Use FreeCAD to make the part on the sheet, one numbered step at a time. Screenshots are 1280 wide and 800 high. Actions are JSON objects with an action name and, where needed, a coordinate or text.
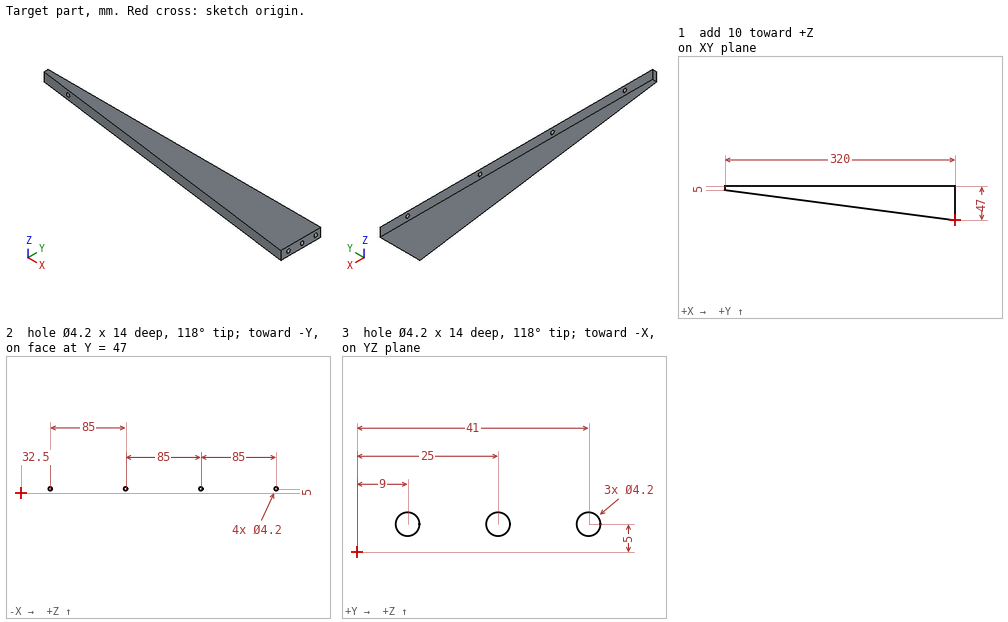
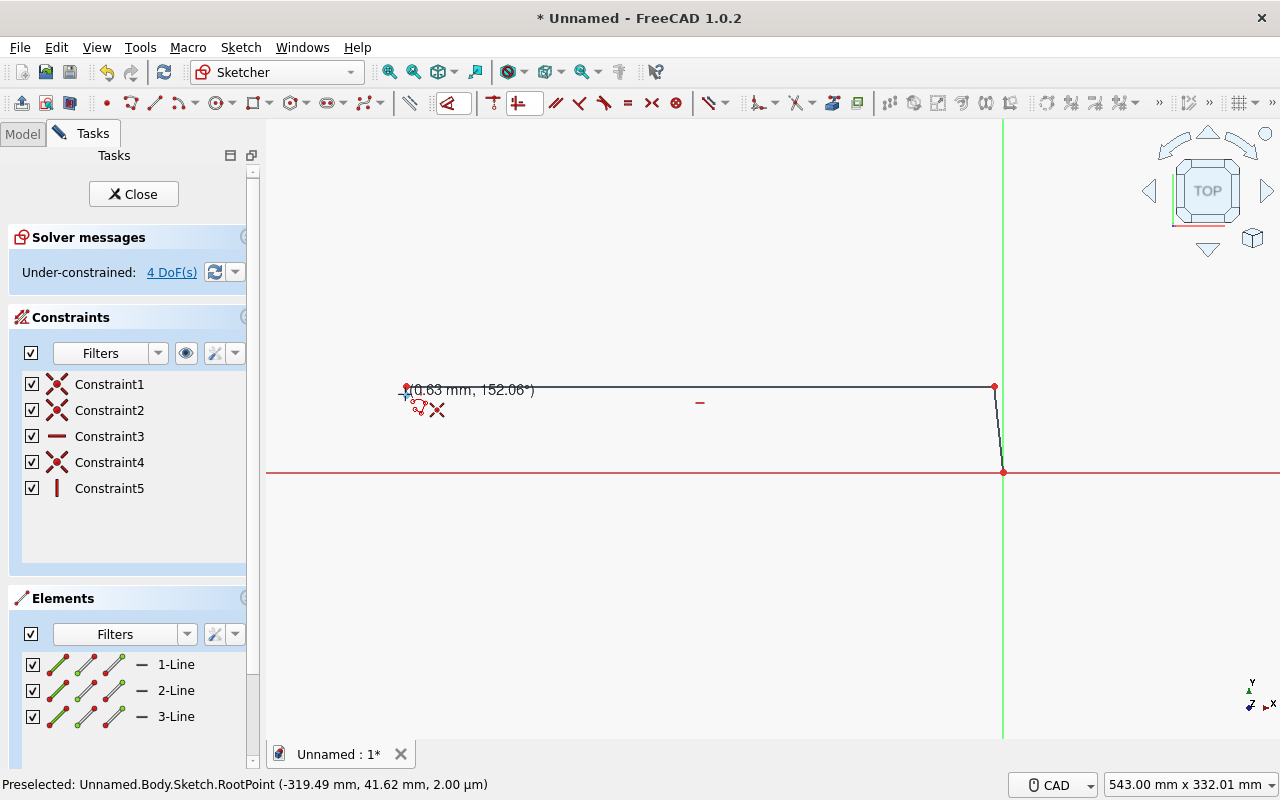
{"action": "left_click", "coordinate": [1003, 473]}
{"action": "key", "text": "Escape"}
{"action": "key", "text": "Escape"}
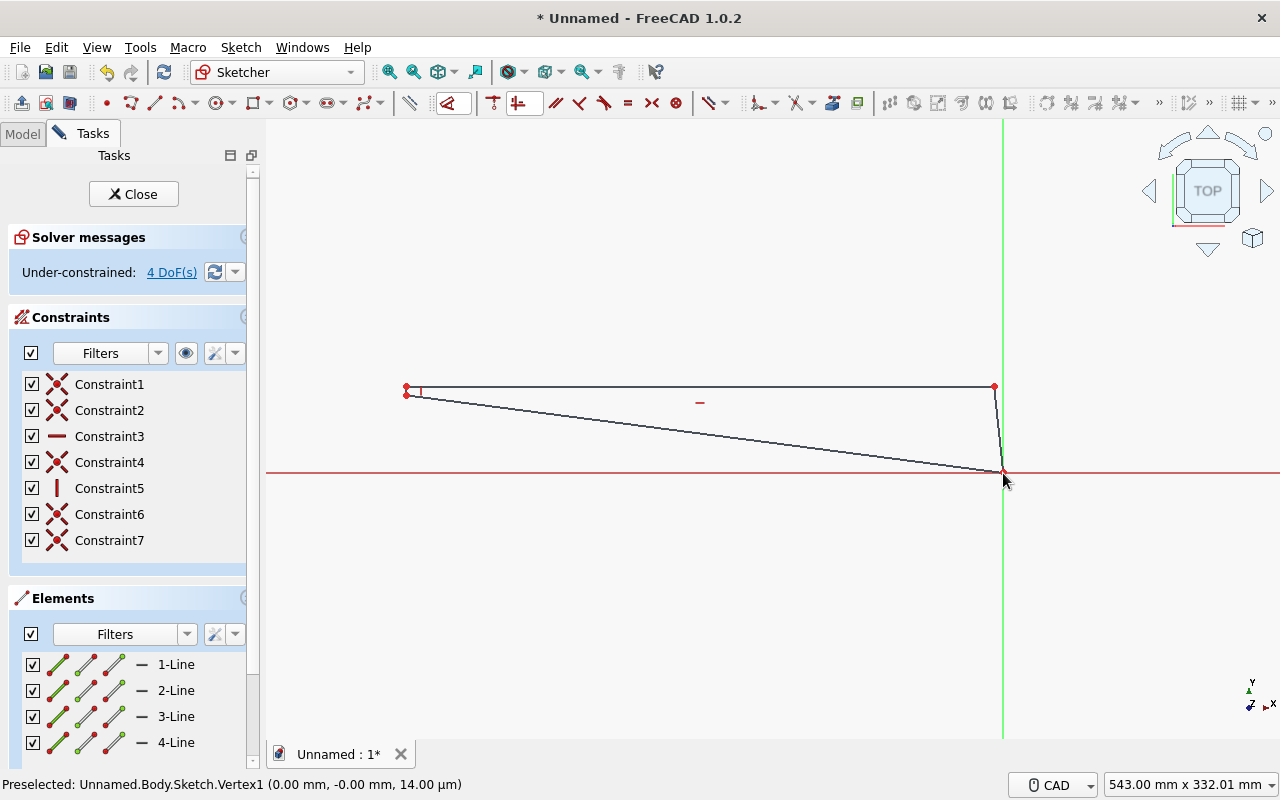
{"action": "left_click", "coordinate": [1001, 447]}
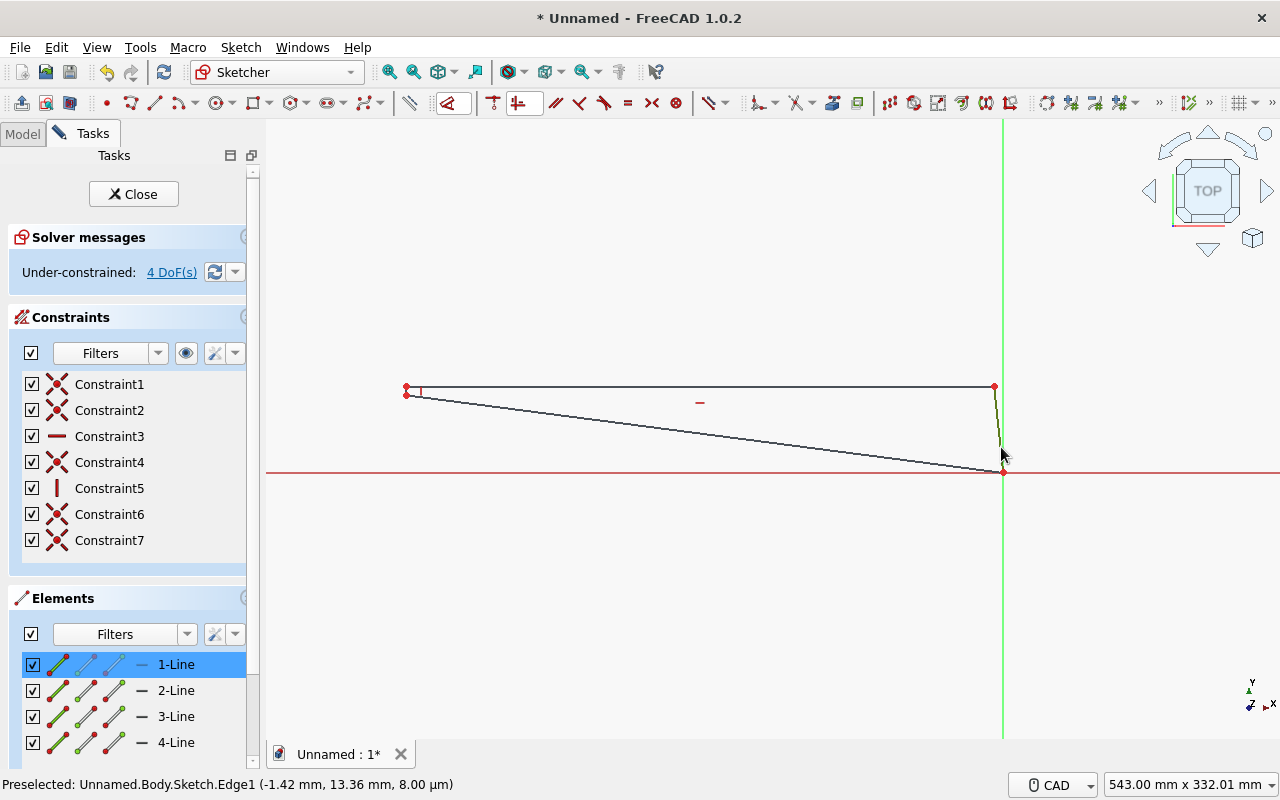
{"action": "key", "text": "v"}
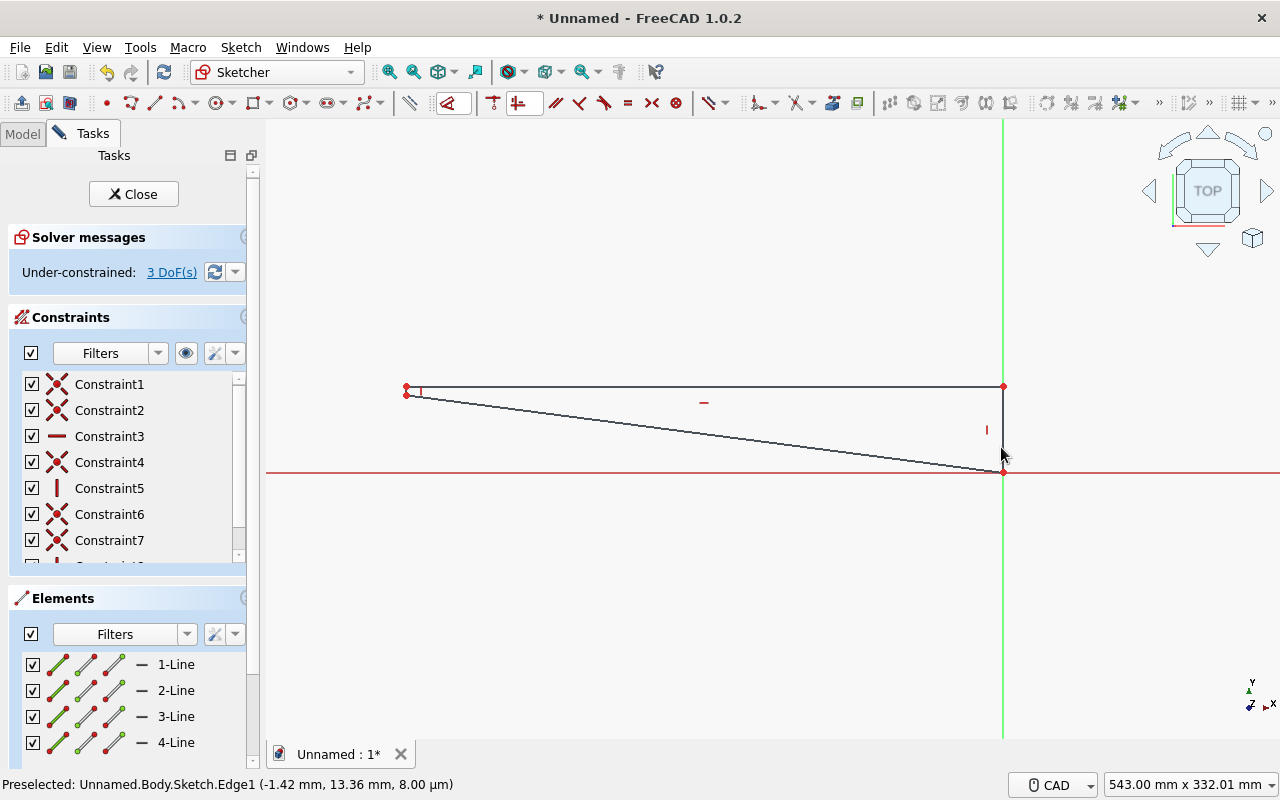
{"action": "key", "text": "d"}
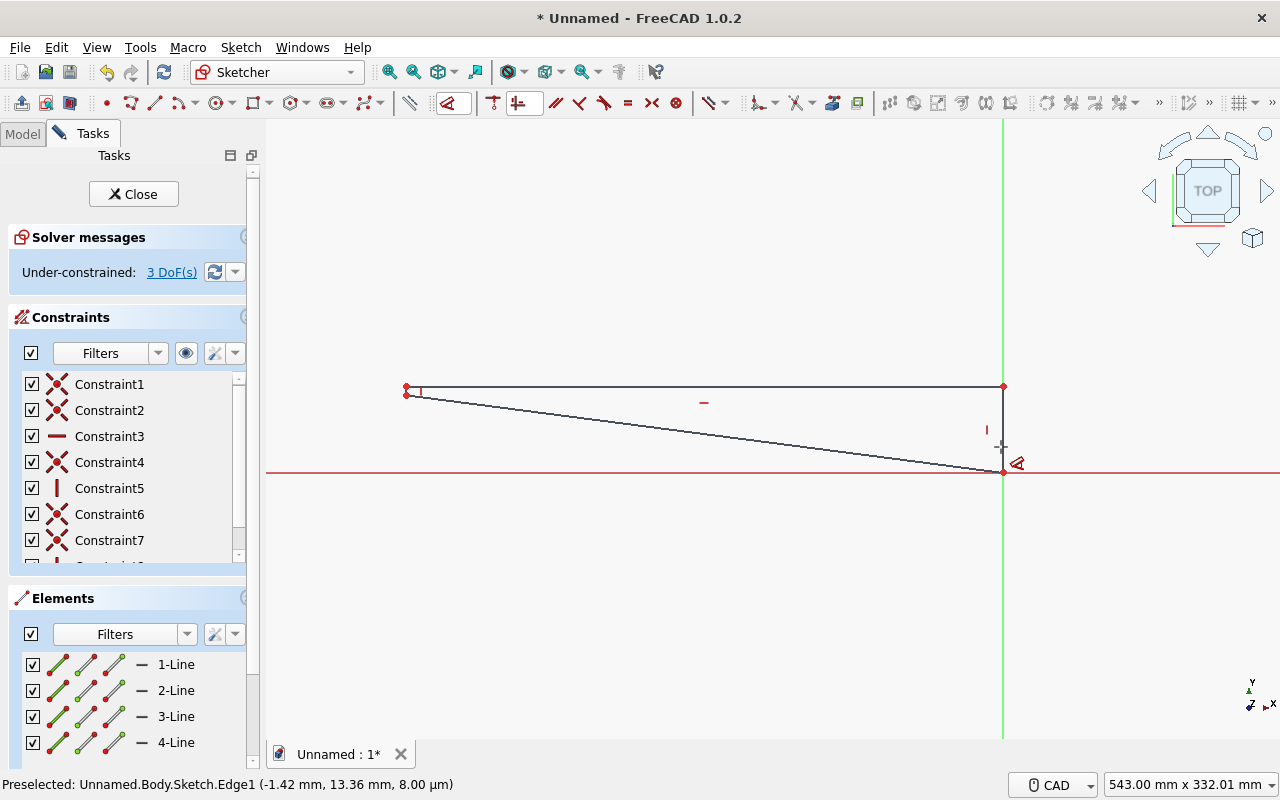
{"action": "scroll", "coordinate": [406, 391], "scroll_direction": "up", "scroll_amount": 8}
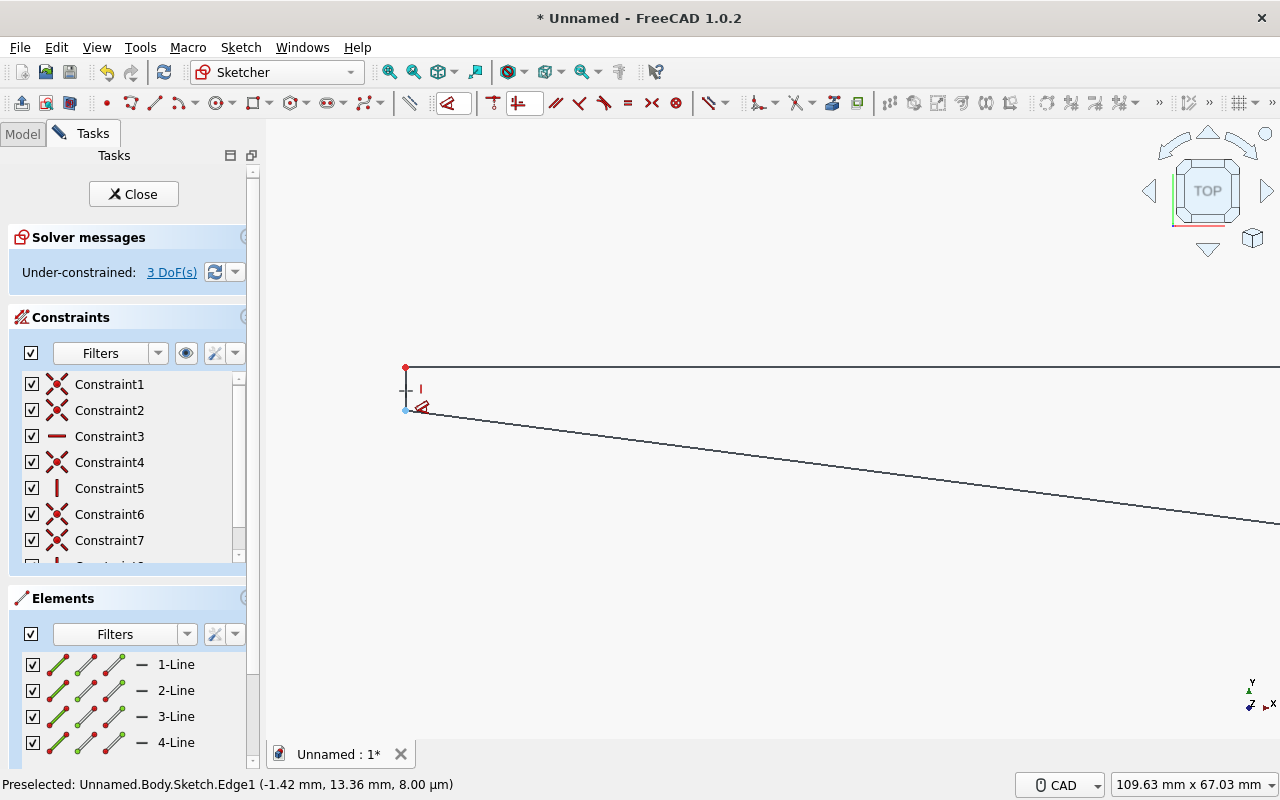
{"action": "left_click", "coordinate": [406, 389]}
{"action": "left_click", "coordinate": [372, 389]}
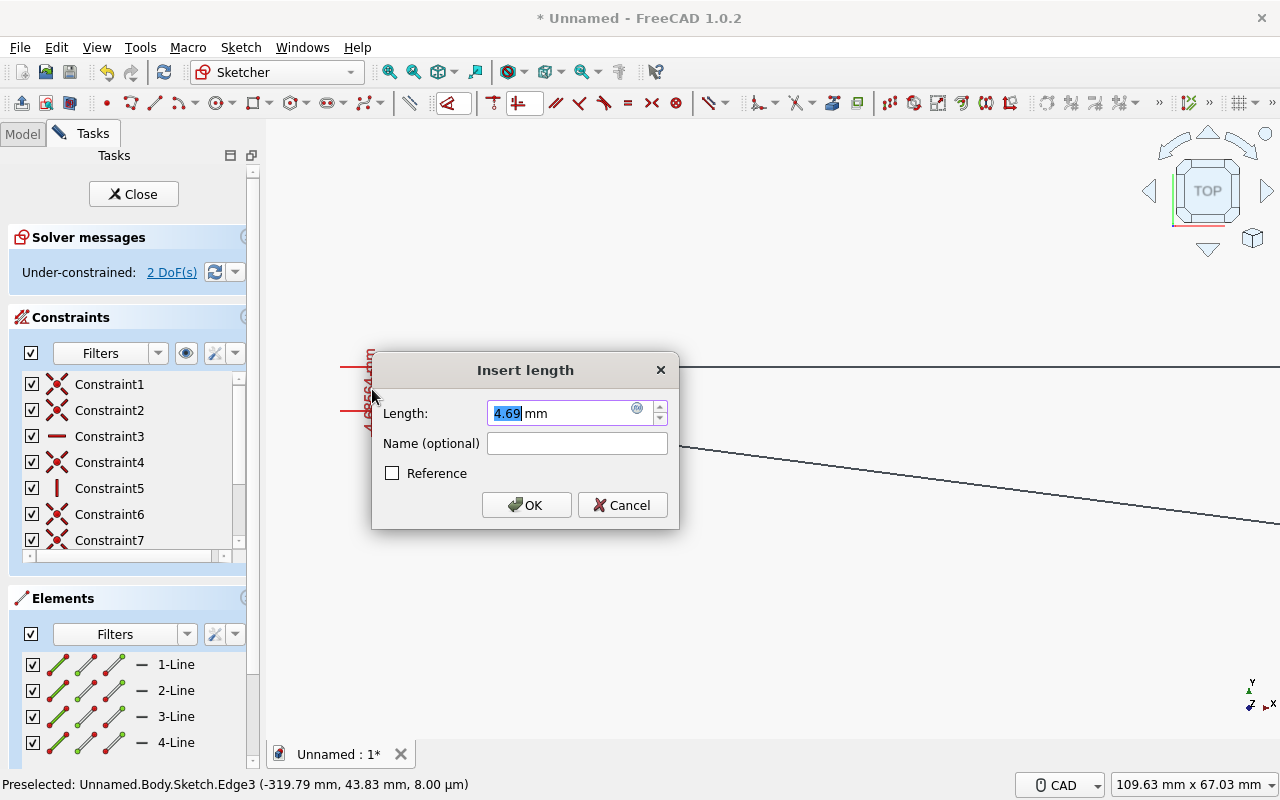
{"action": "type", "text": "5"}
{"action": "key", "text": "Return"}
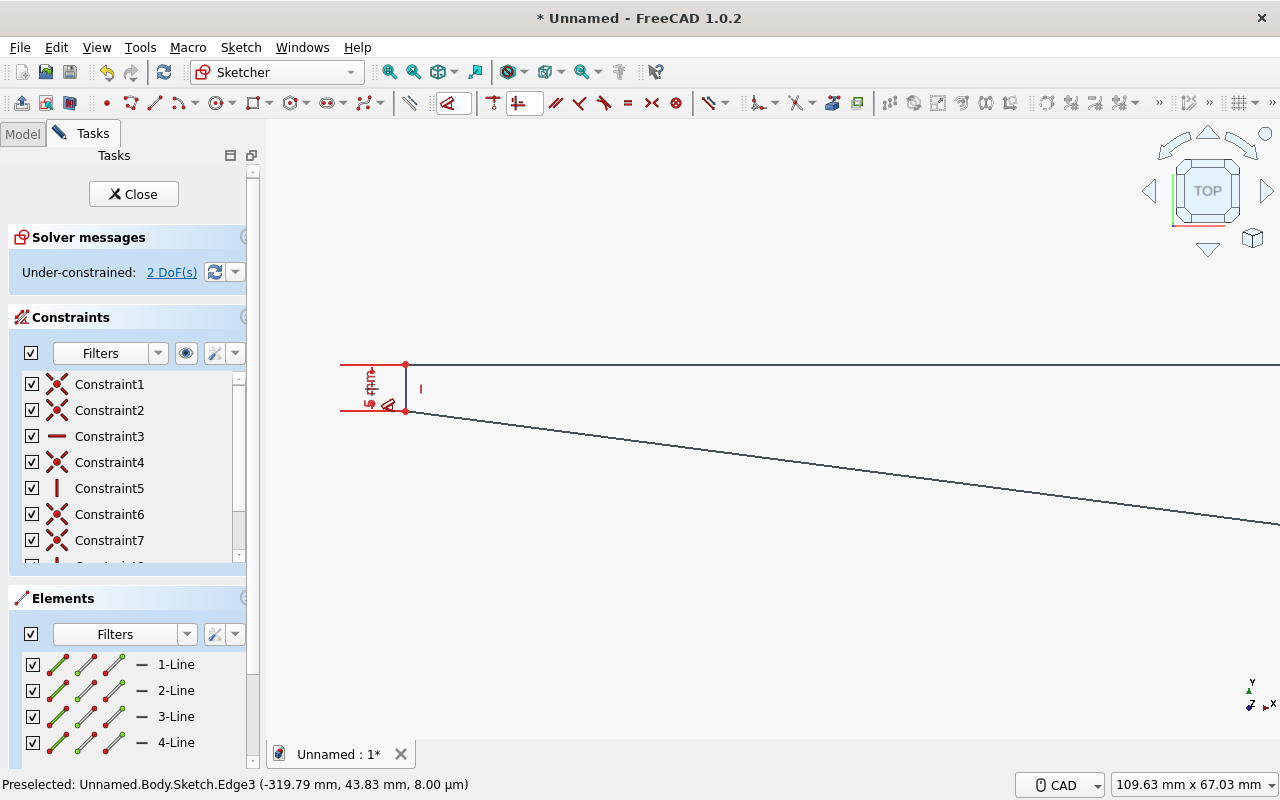
{"action": "scroll", "coordinate": [406, 391], "scroll_direction": "down", "scroll_amount": 8}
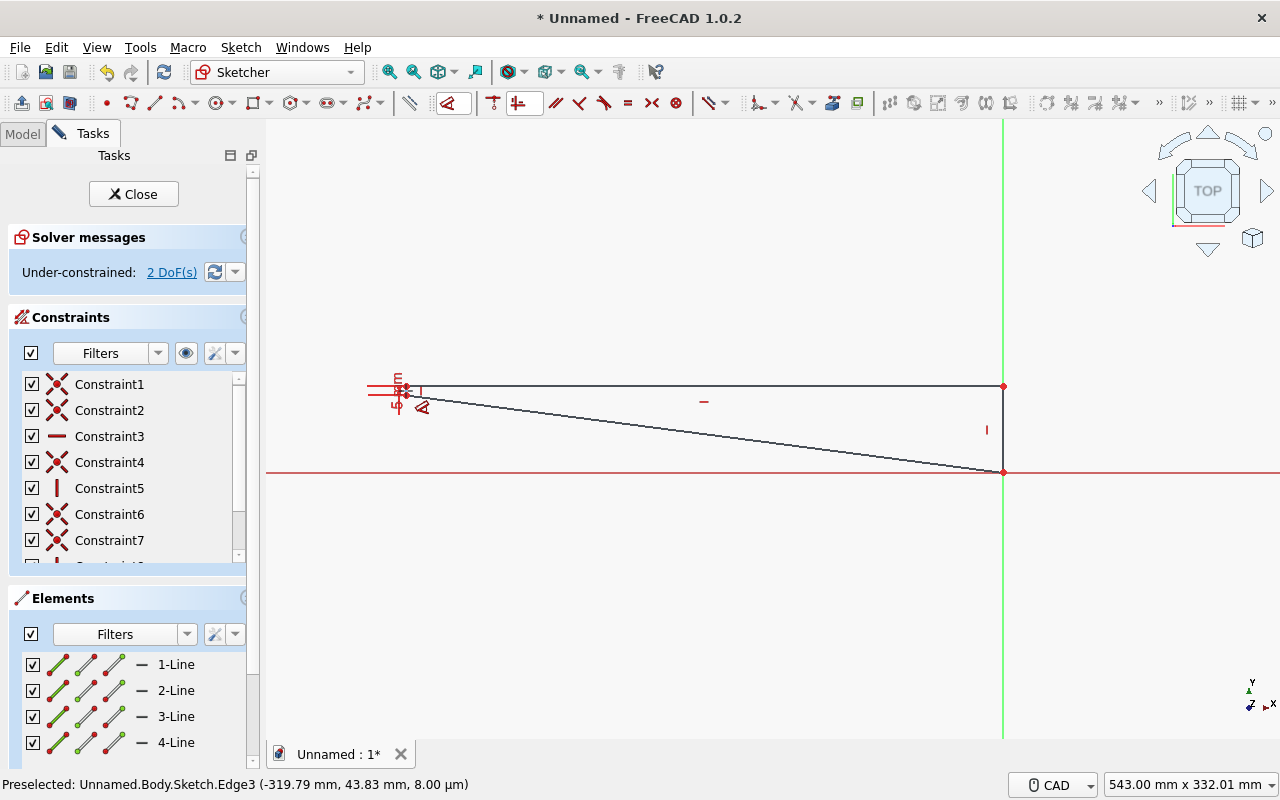
{"action": "left_click", "coordinate": [1003, 447]}
{"action": "left_click", "coordinate": [1037, 430]}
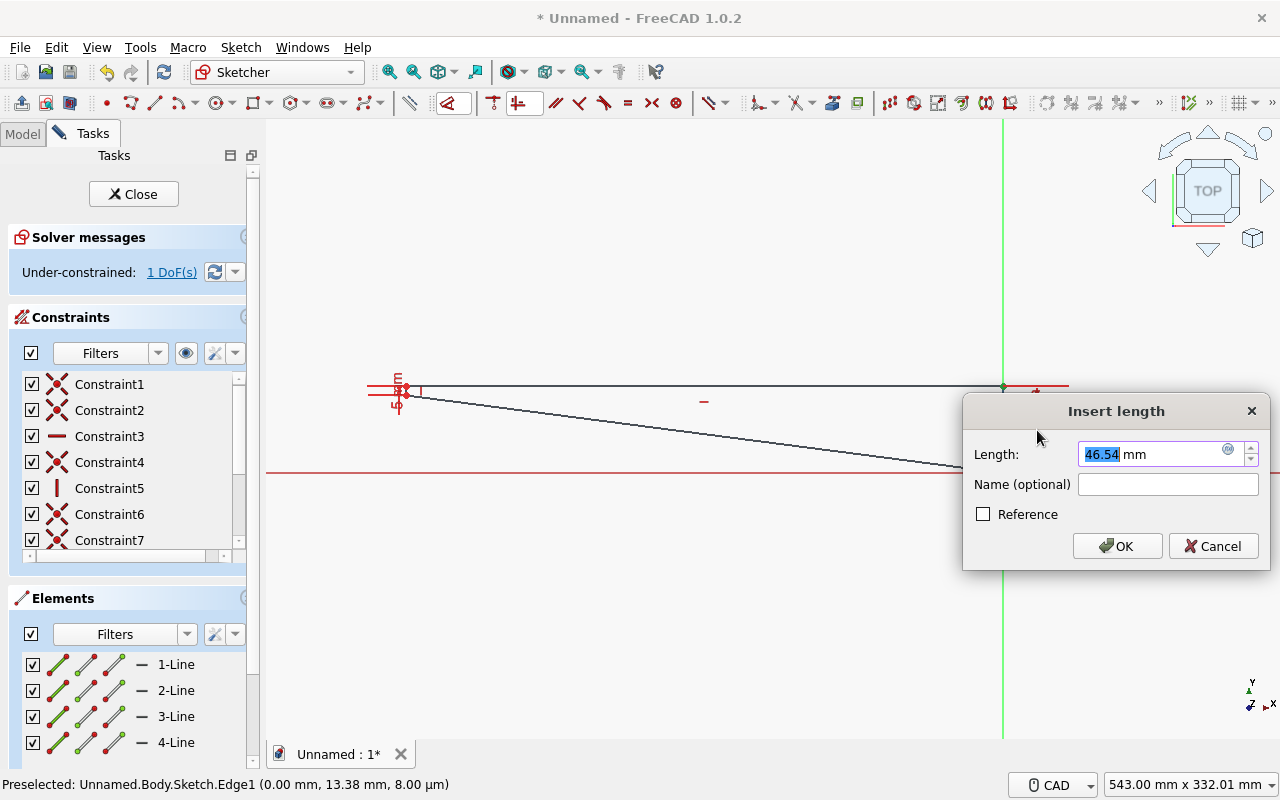
{"action": "type", "text": "47"}
{"action": "key", "text": "Return"}